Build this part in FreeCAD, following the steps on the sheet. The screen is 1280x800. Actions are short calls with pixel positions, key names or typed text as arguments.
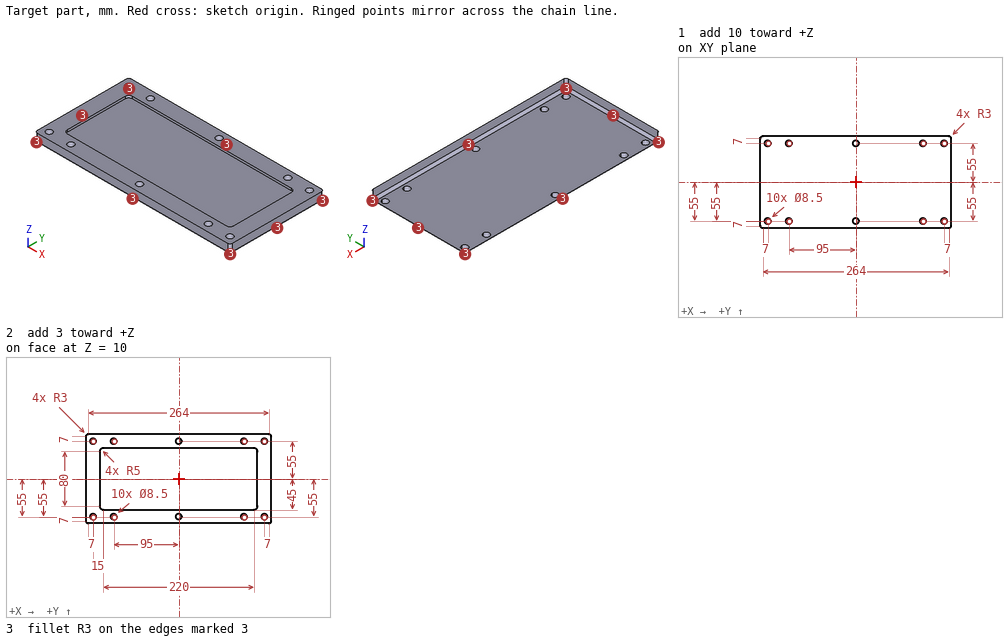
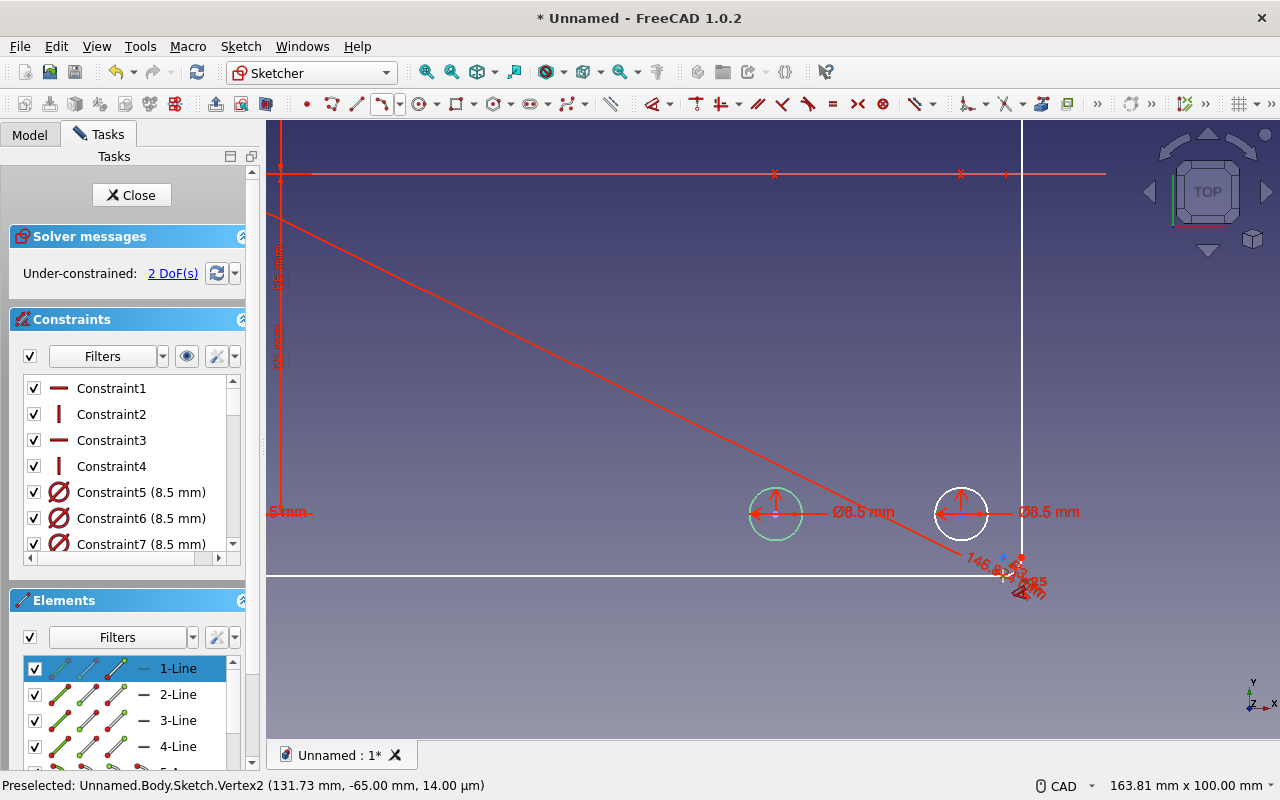
click(961, 514)
click(982, 610)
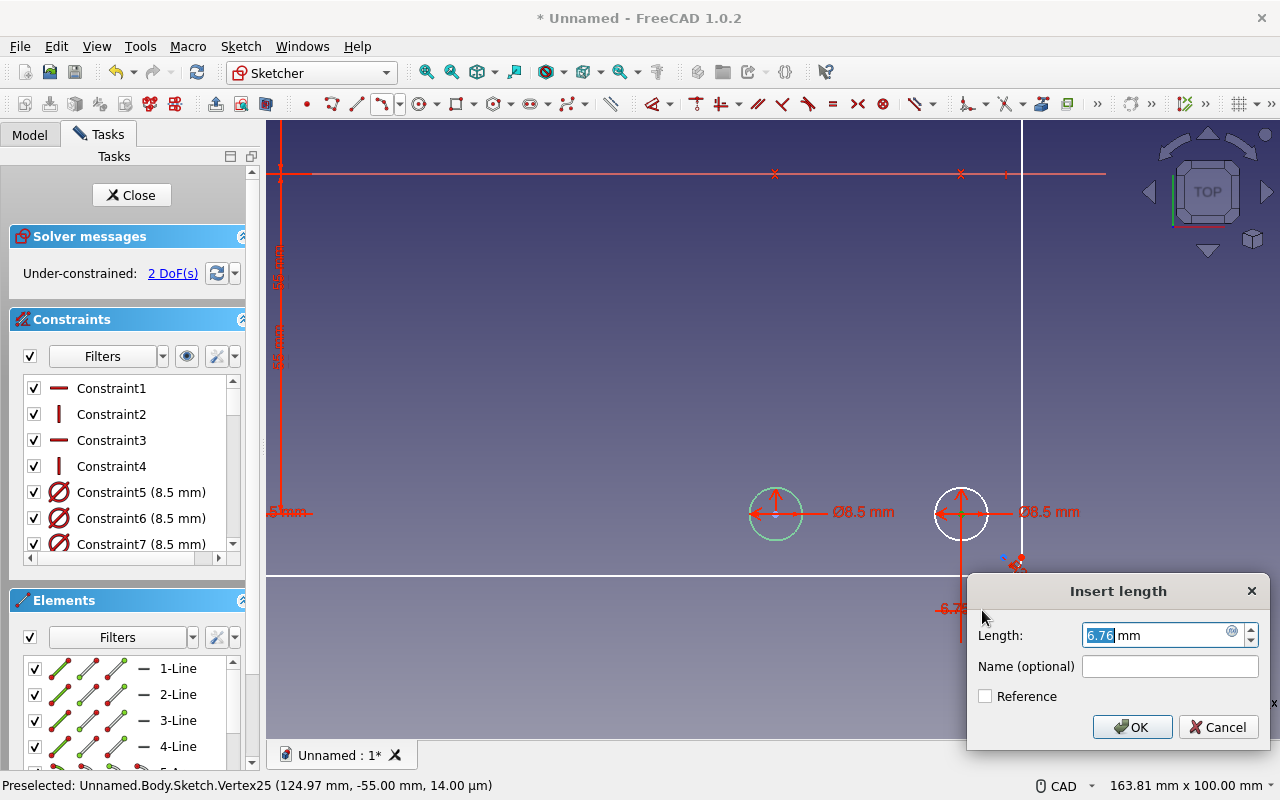
text(7)
key(Return)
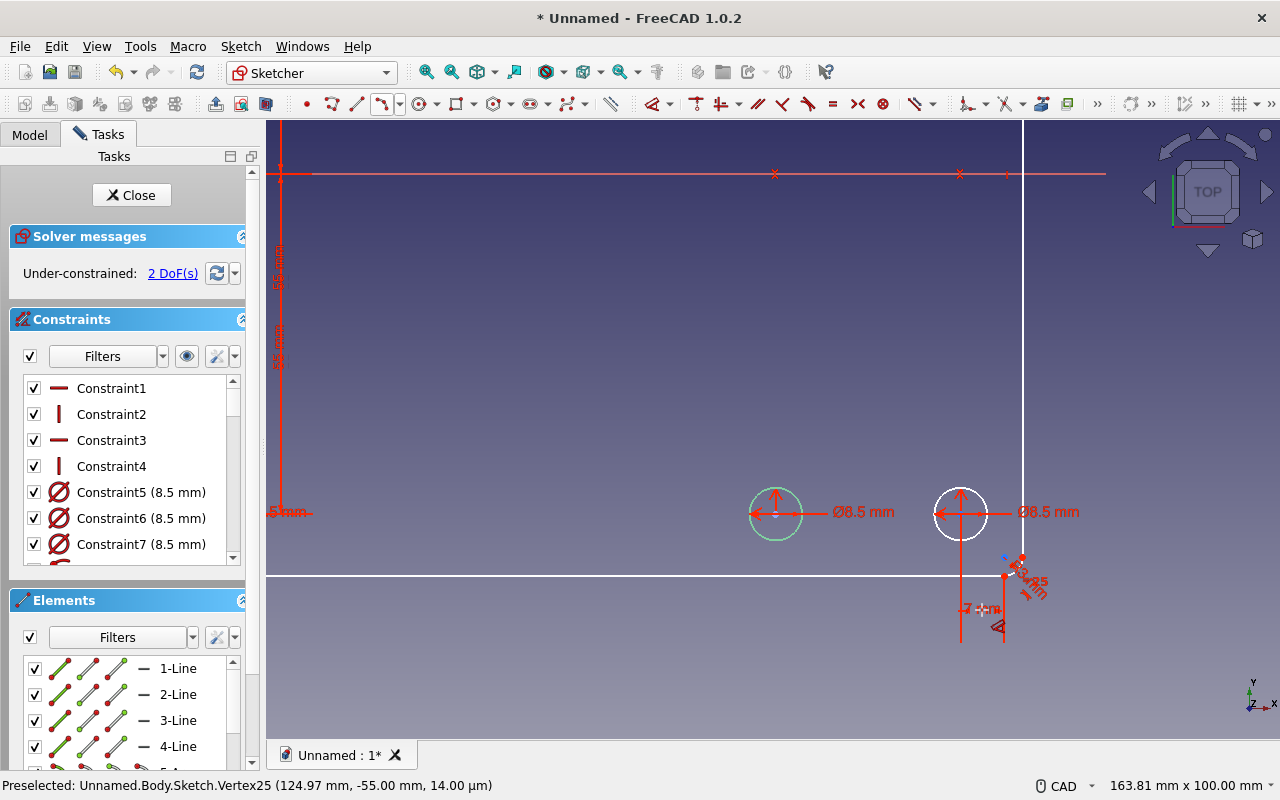
scroll(1005, 578, down, 5)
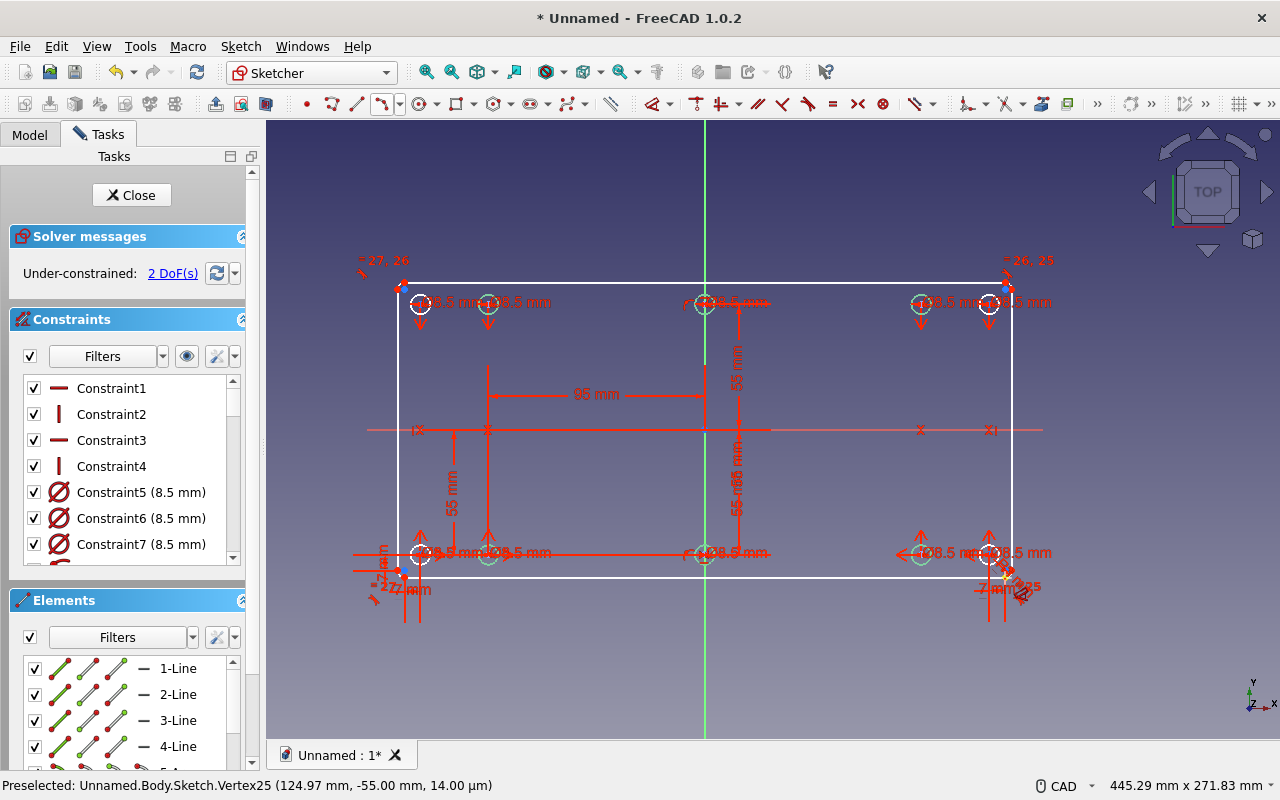
scroll(398, 289, up, 5)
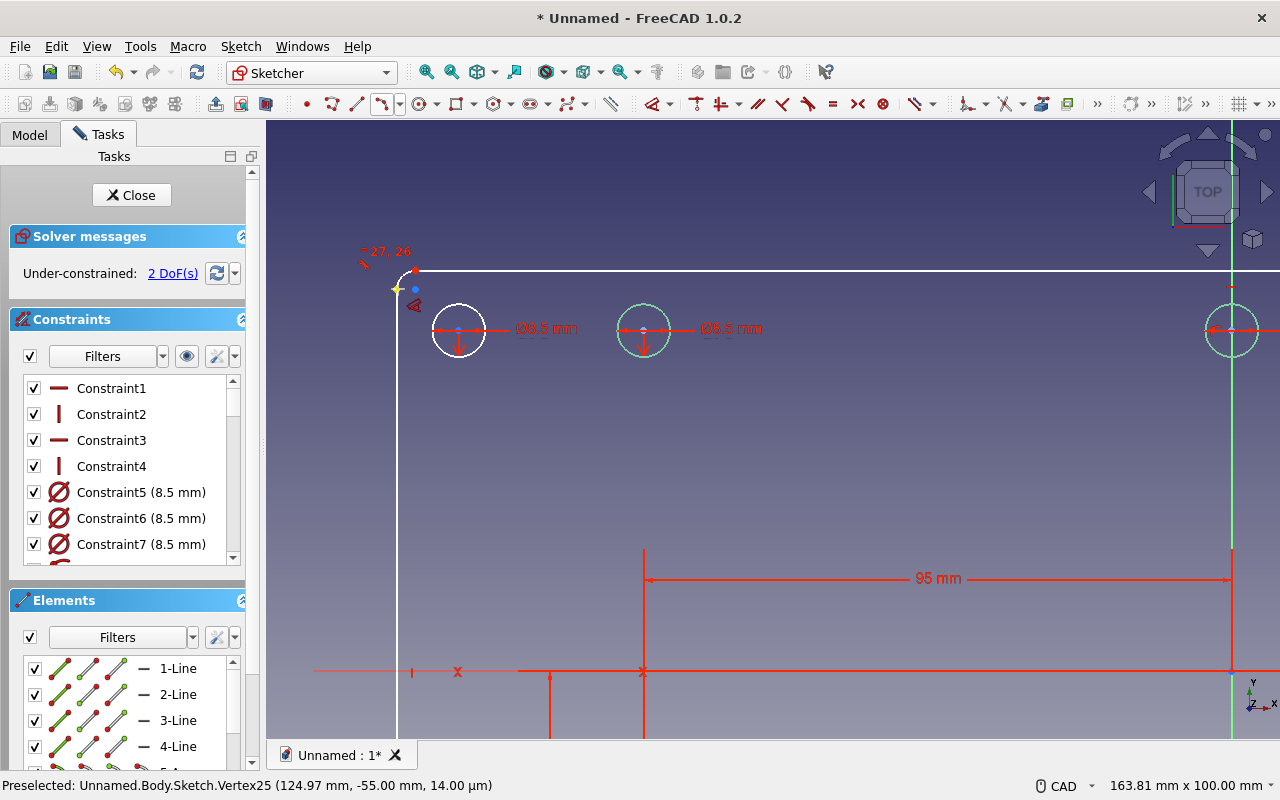
click(397, 289)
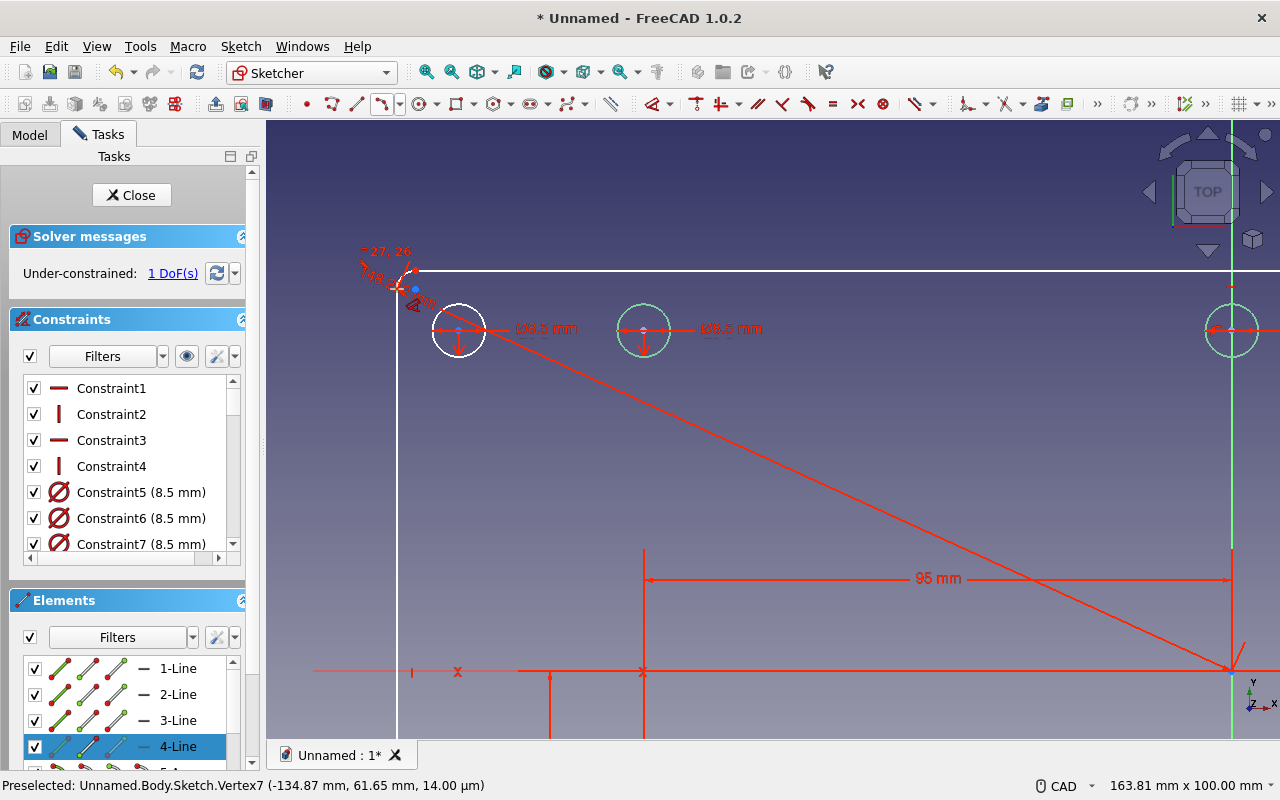
click(459, 331)
click(363, 310)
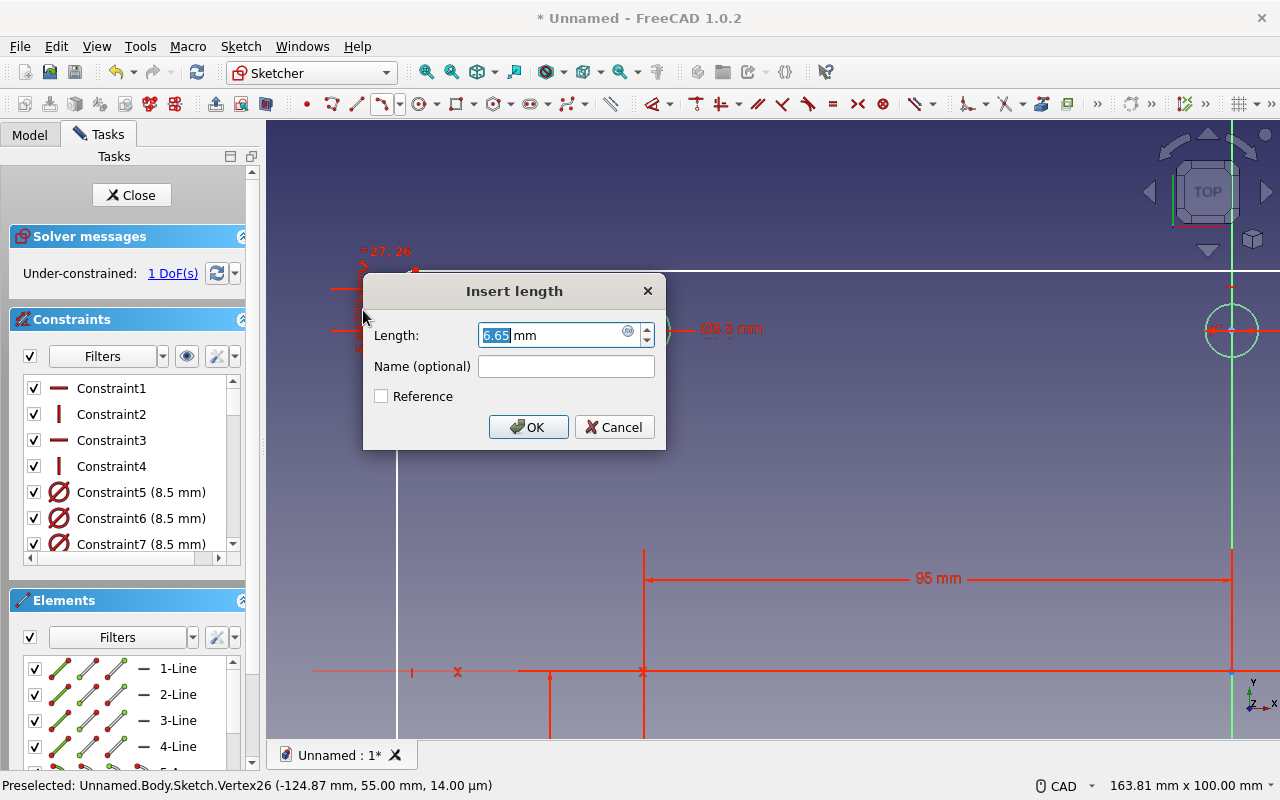
text(7)
key(Return)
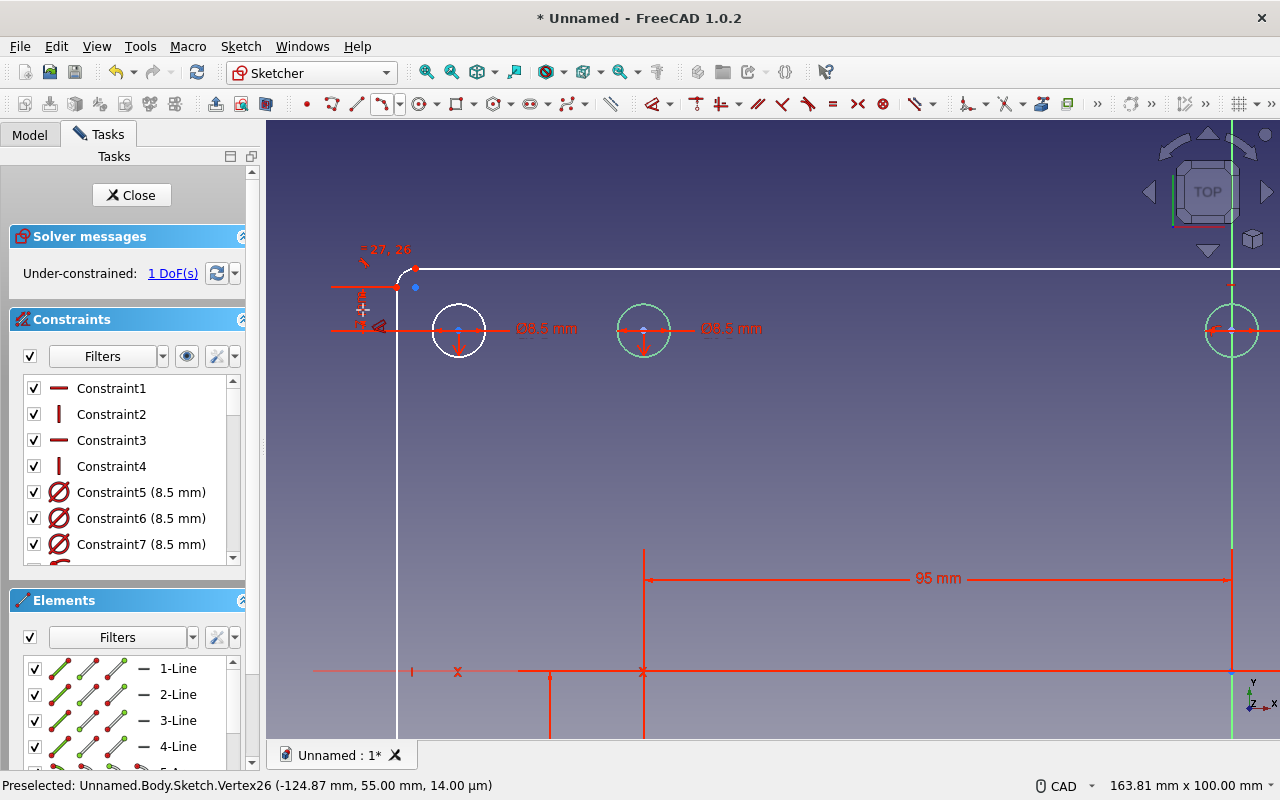
scroll(398, 289, down, 5)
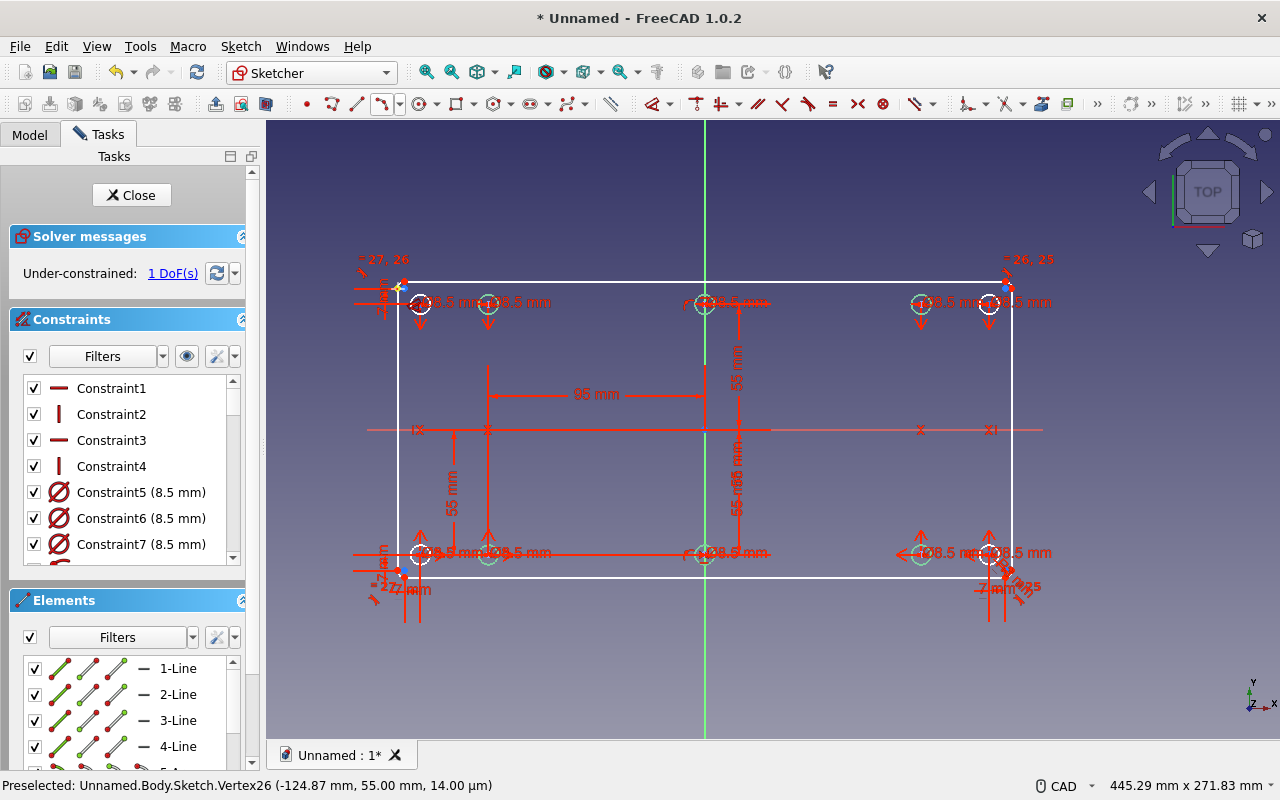
click(585, 578)
click(567, 612)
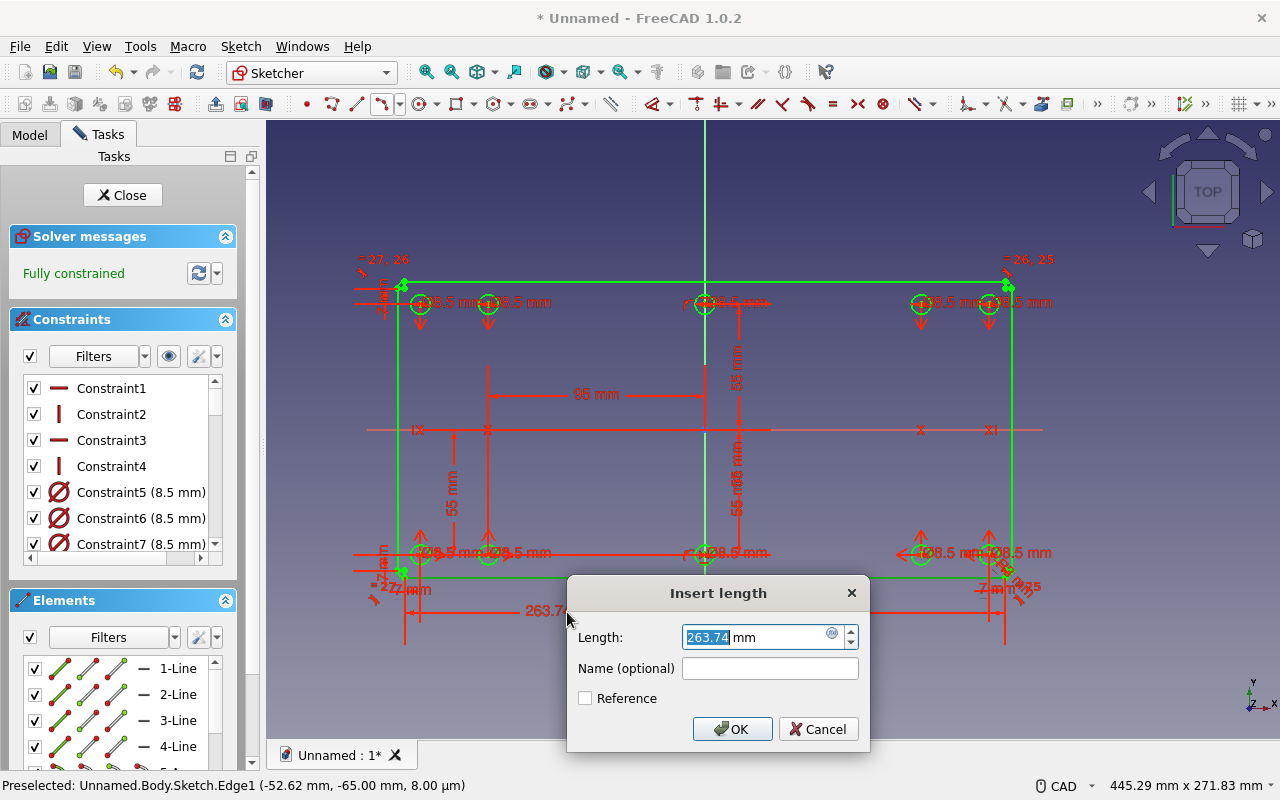
text(264)
key(Return)
key(Escape)